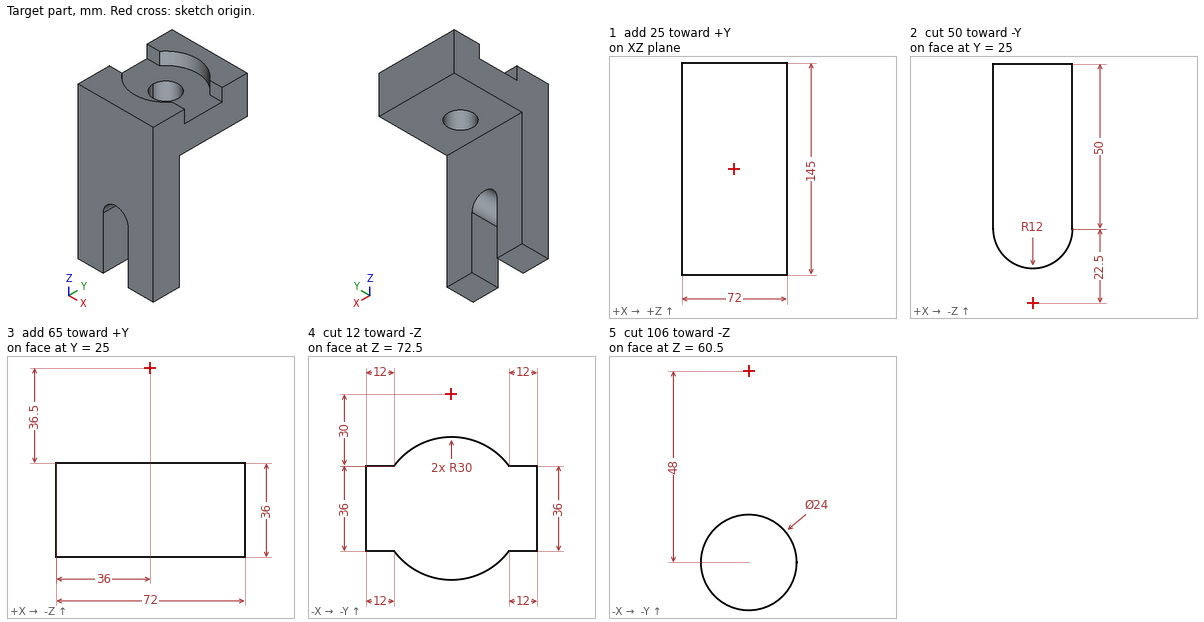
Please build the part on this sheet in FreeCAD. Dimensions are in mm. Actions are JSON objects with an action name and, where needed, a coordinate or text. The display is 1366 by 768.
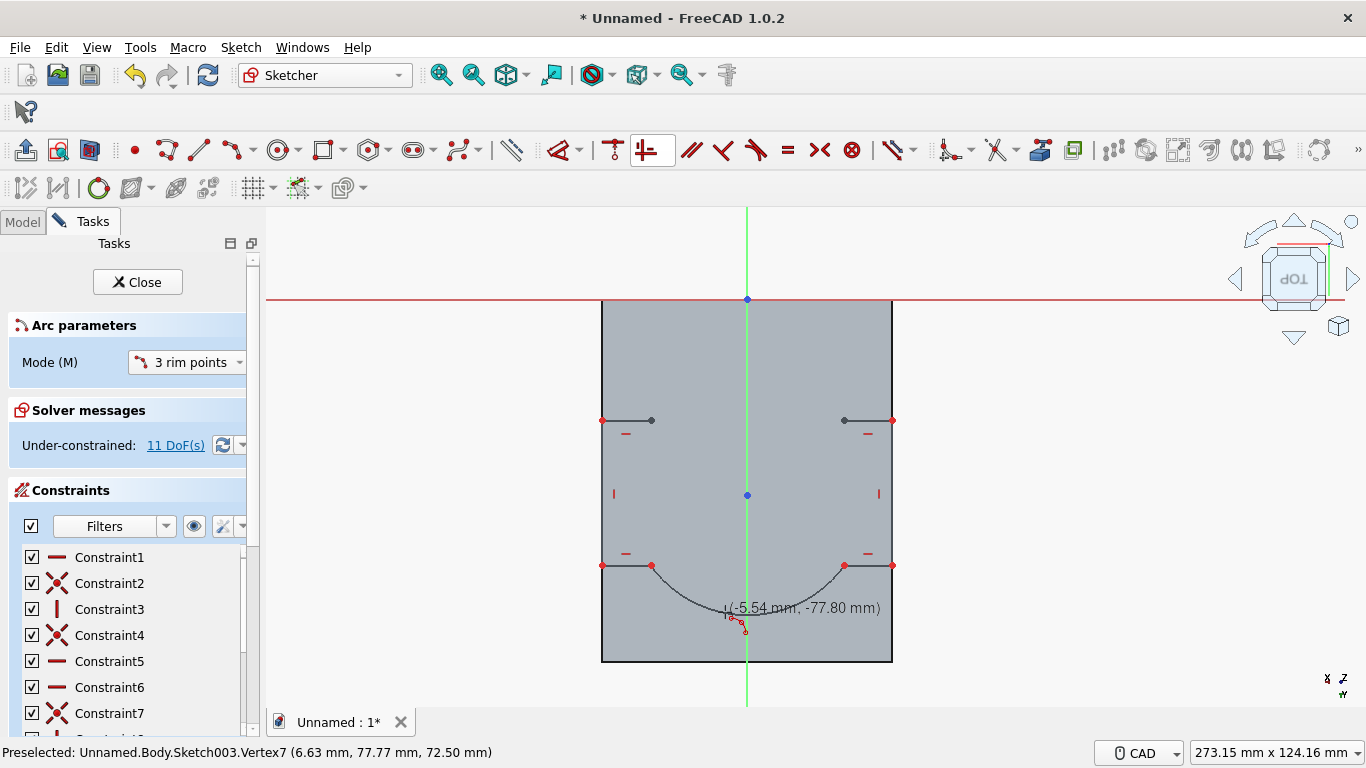
{"action": "left_click", "coordinate": [844, 421]}
{"action": "left_click", "coordinate": [651, 421]}
{"action": "left_click", "coordinate": [770, 374]}
{"action": "key", "text": "Escape"}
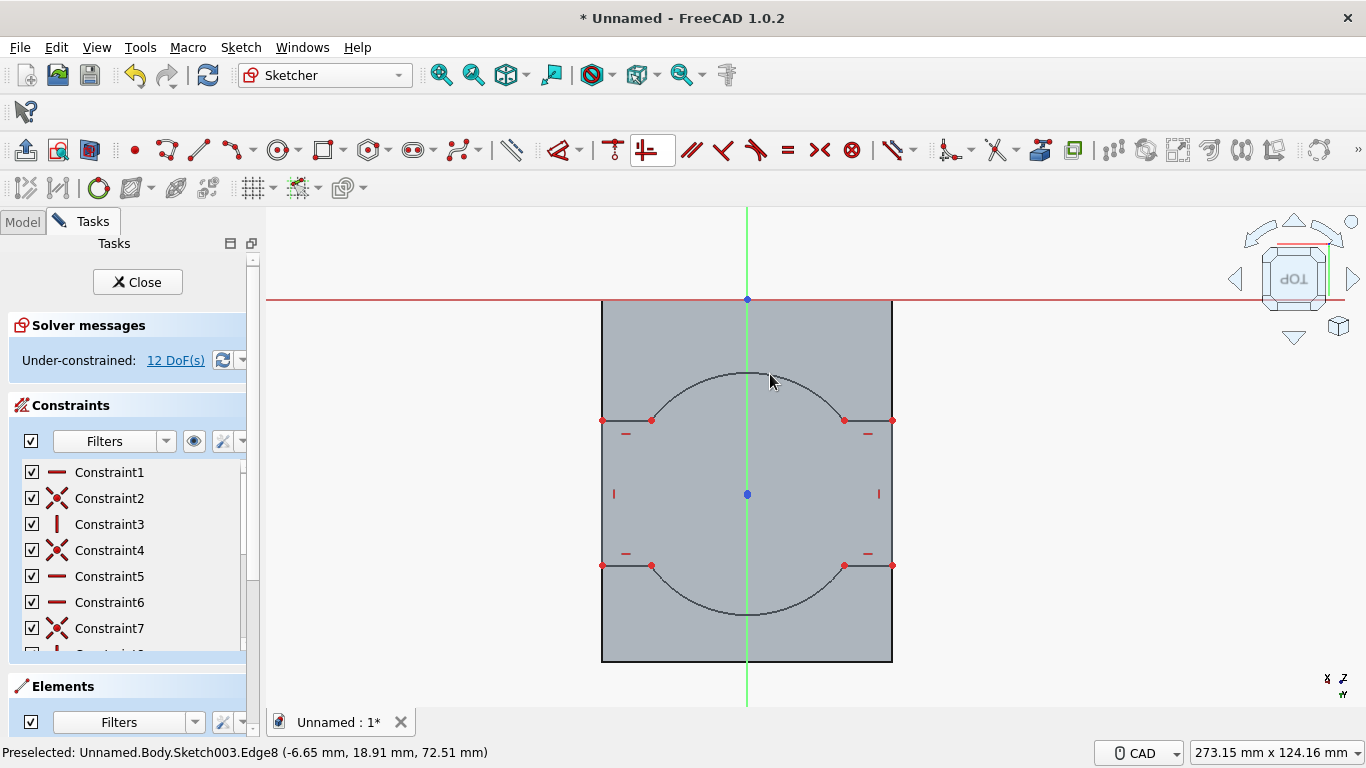
{"action": "left_click", "coordinate": [704, 607]}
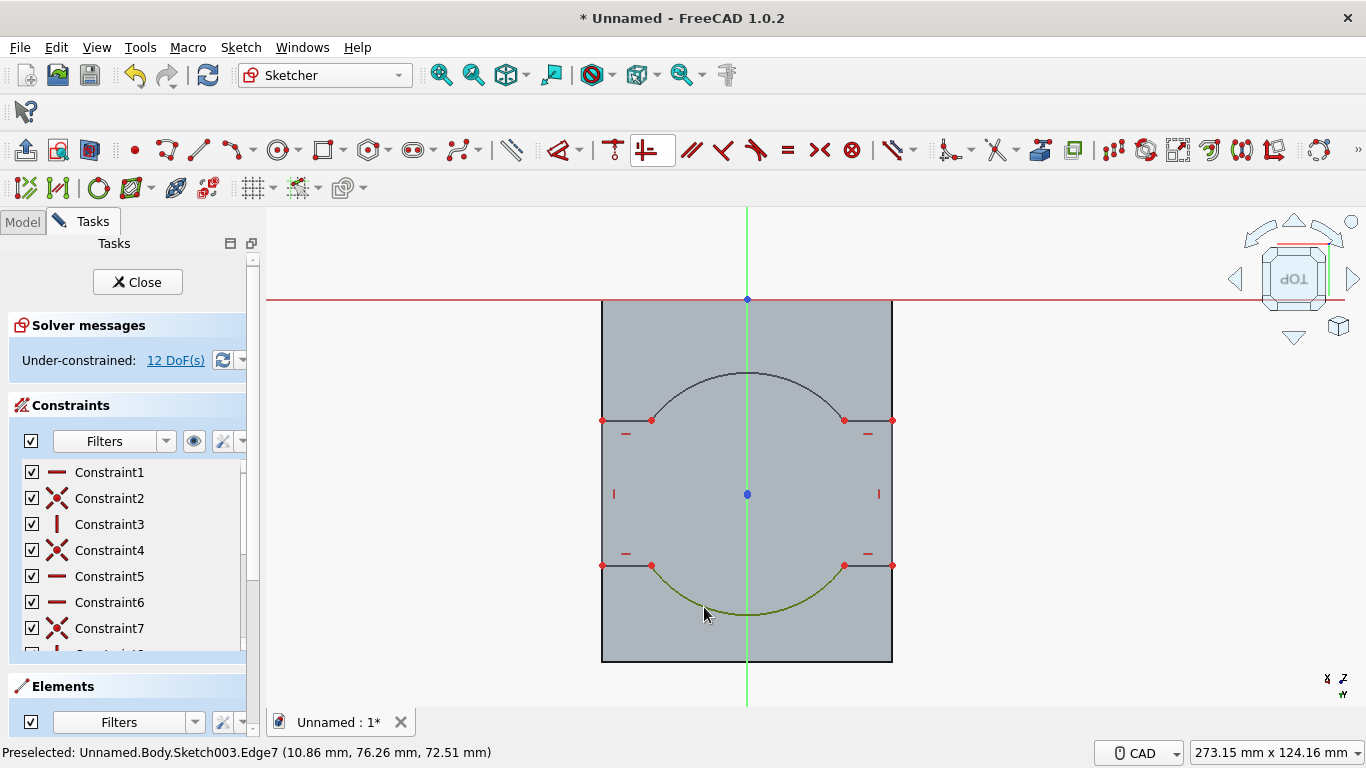
{"action": "left_click", "coordinate": [791, 381]}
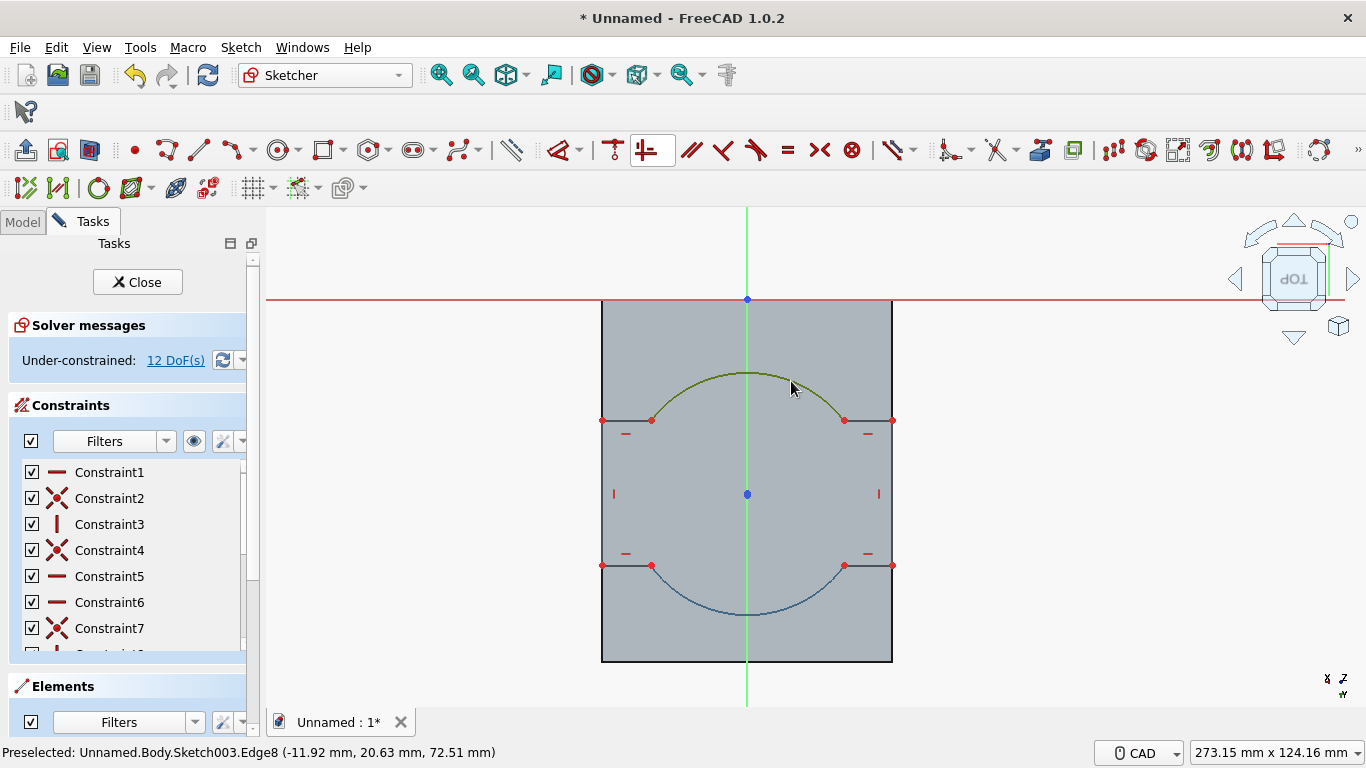
{"action": "left_click", "coordinate": [614, 150]}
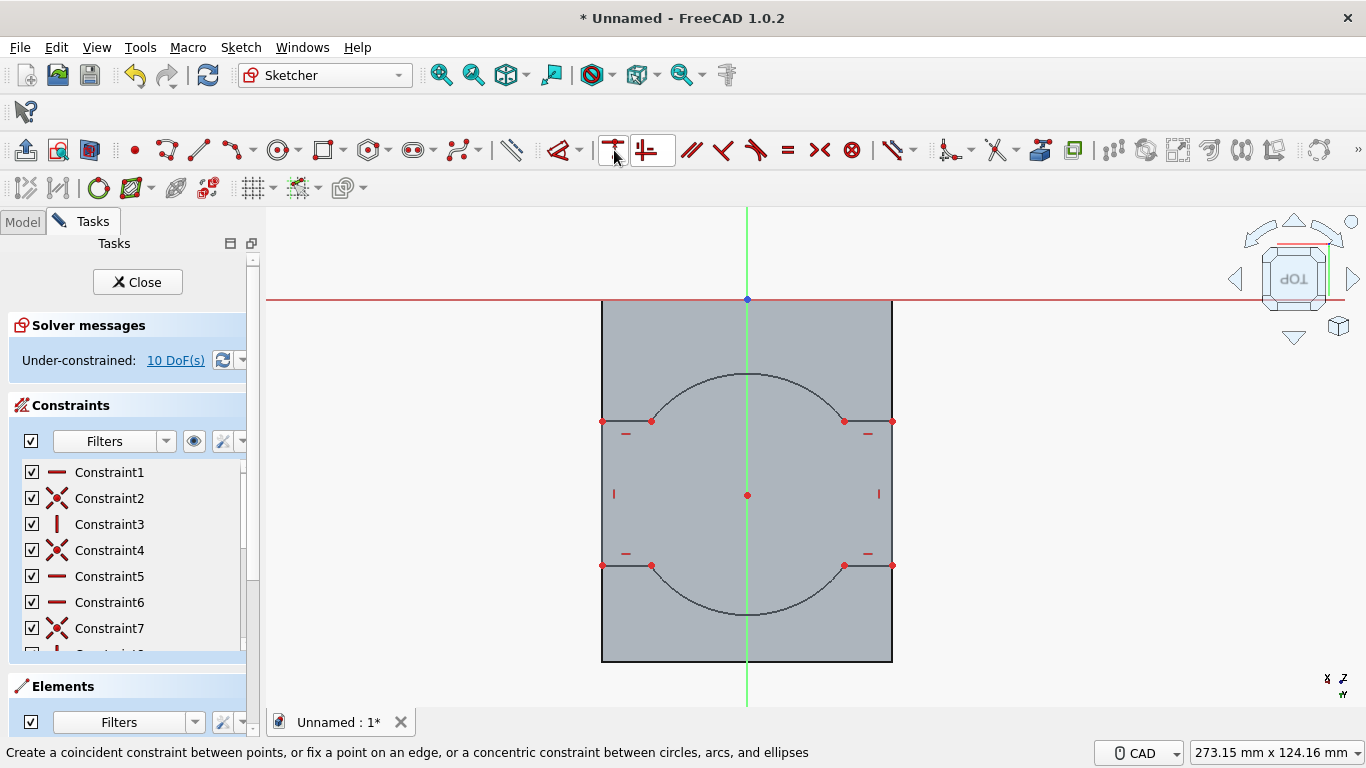
{"action": "left_click", "coordinate": [704, 607]}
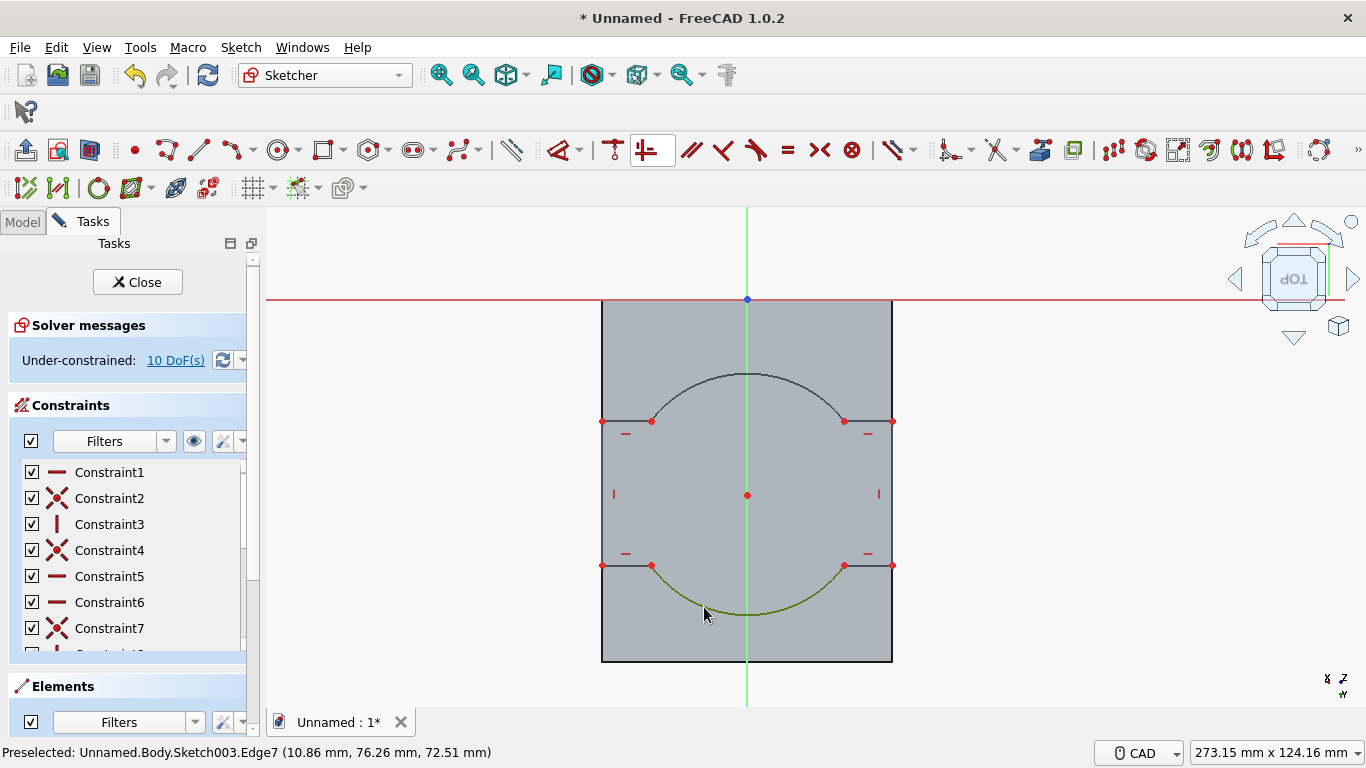
{"action": "left_click", "coordinate": [791, 382]}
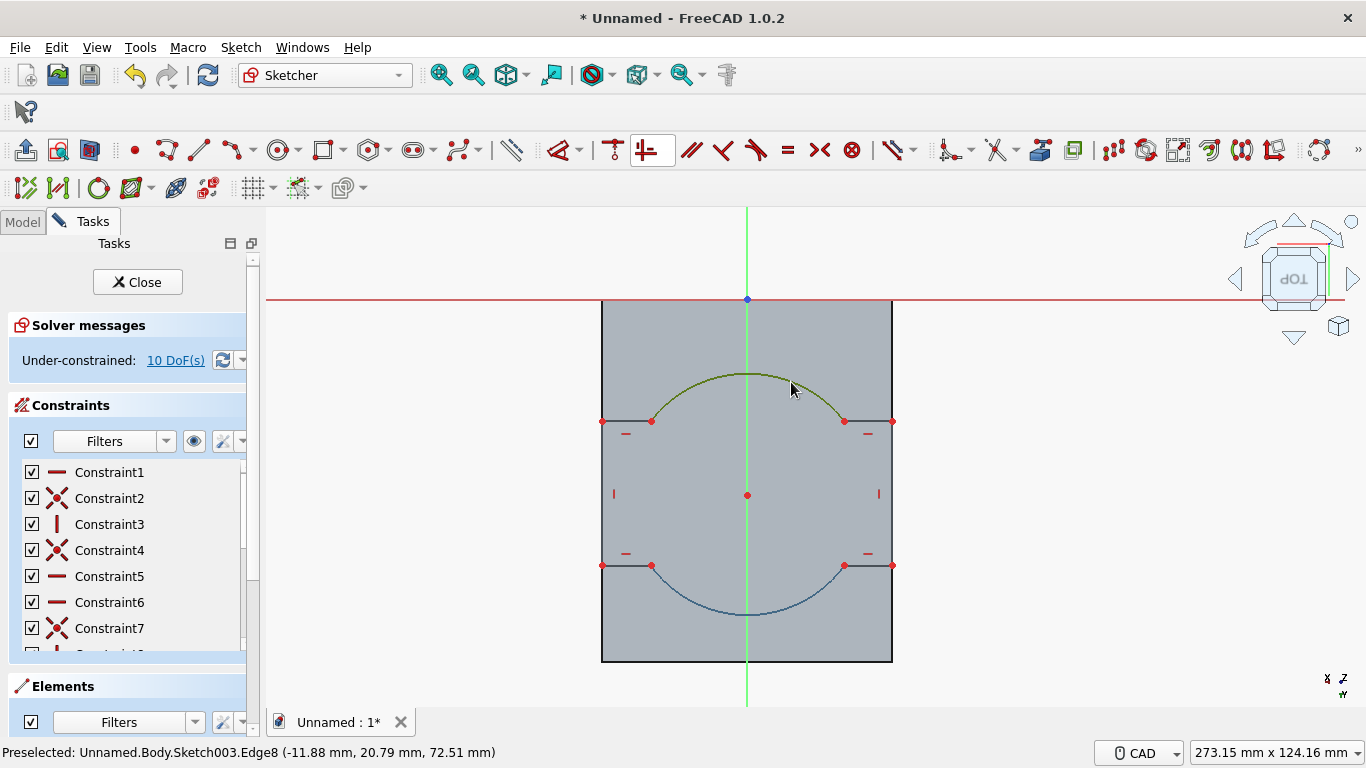
{"action": "left_click", "coordinate": [788, 150]}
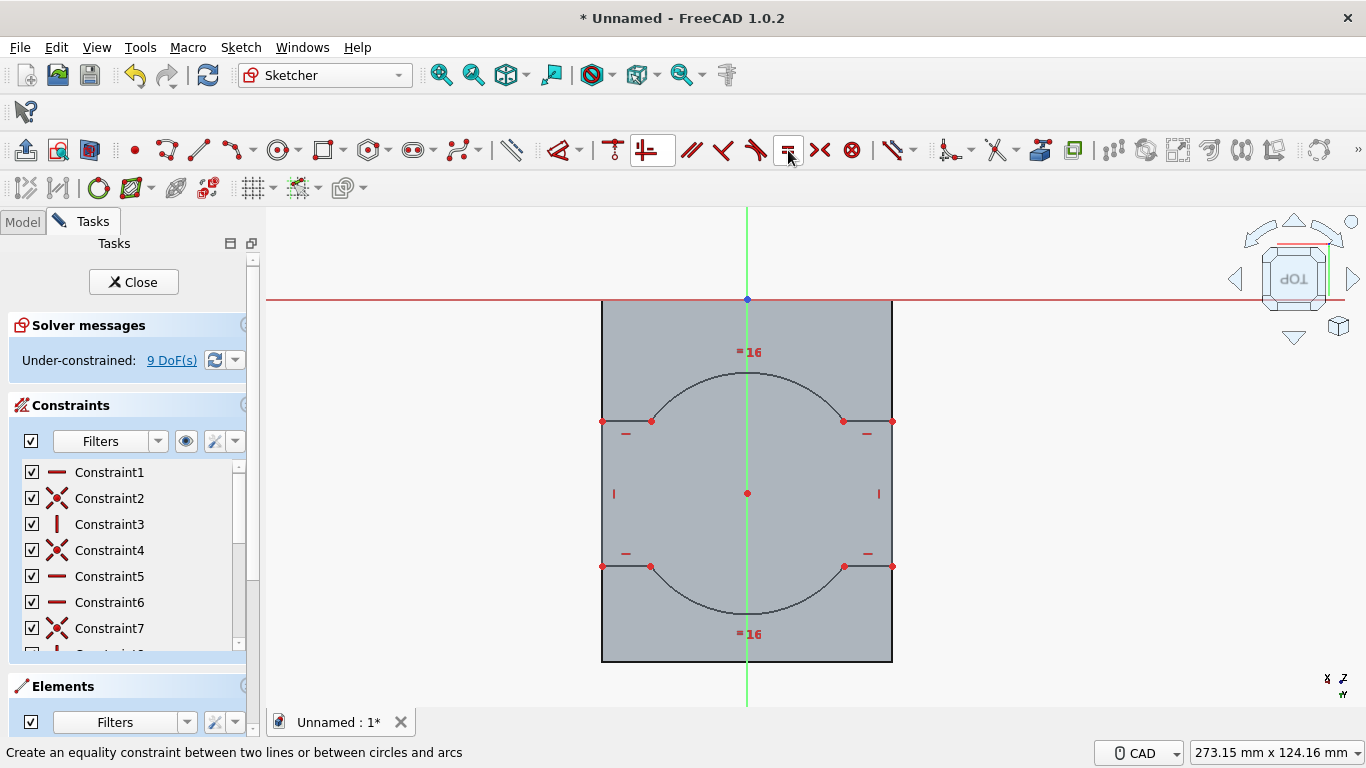
{"action": "left_click", "coordinate": [747, 494]}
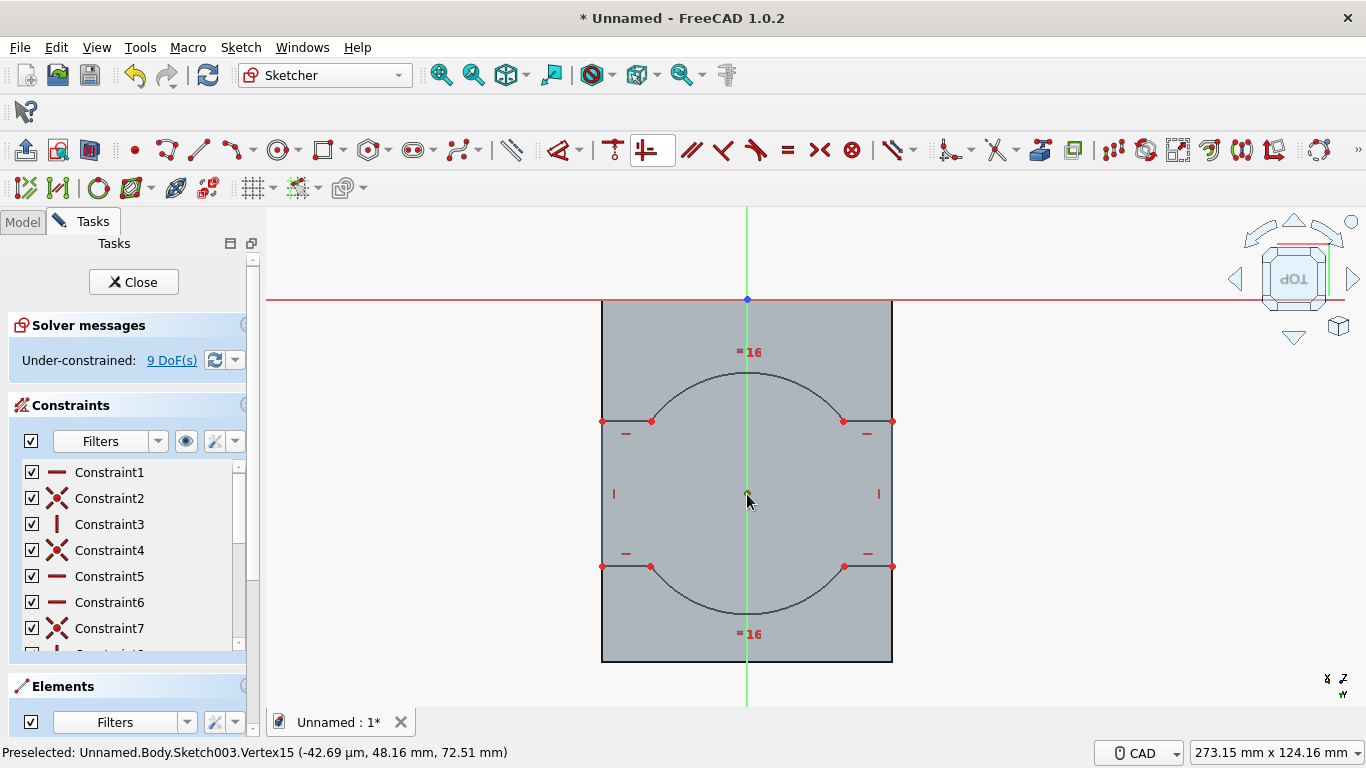
{"action": "left_click", "coordinate": [747, 647]}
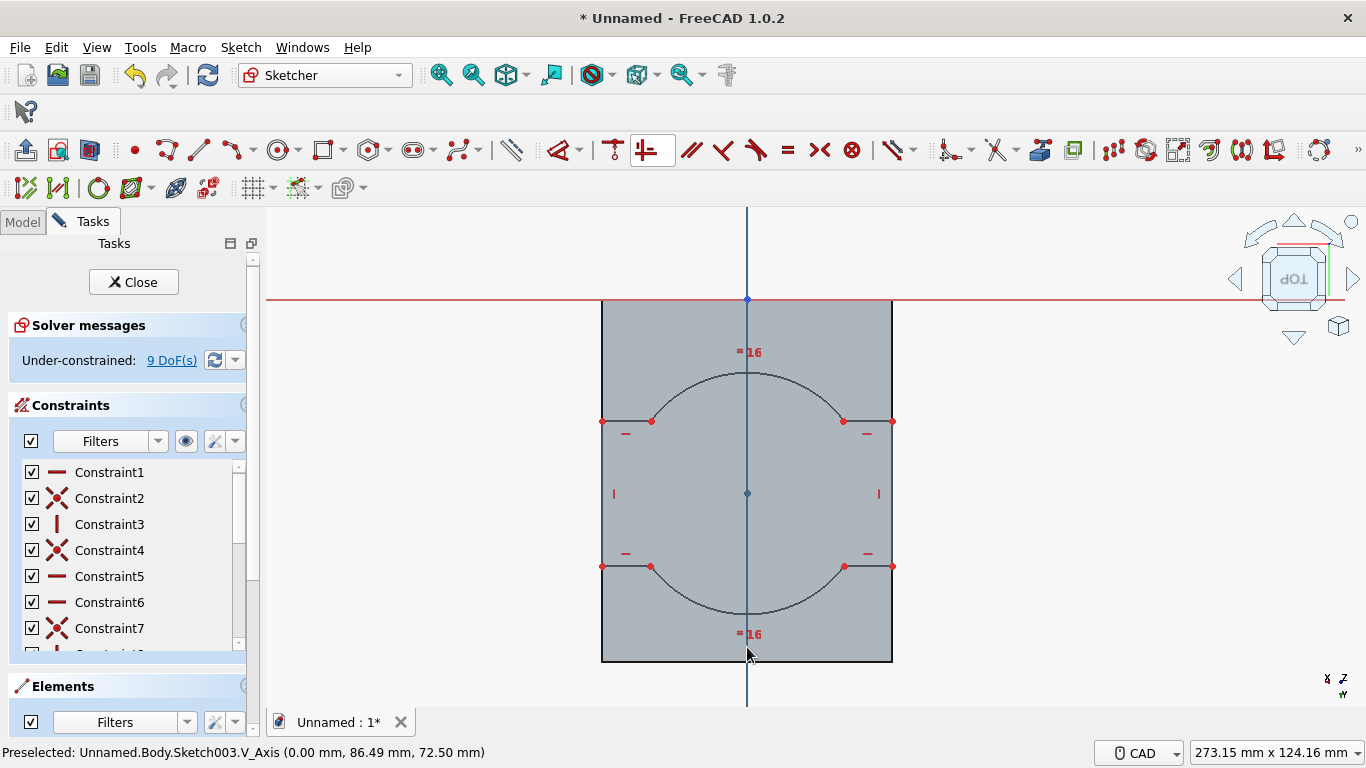
{"action": "left_click", "coordinate": [614, 150]}